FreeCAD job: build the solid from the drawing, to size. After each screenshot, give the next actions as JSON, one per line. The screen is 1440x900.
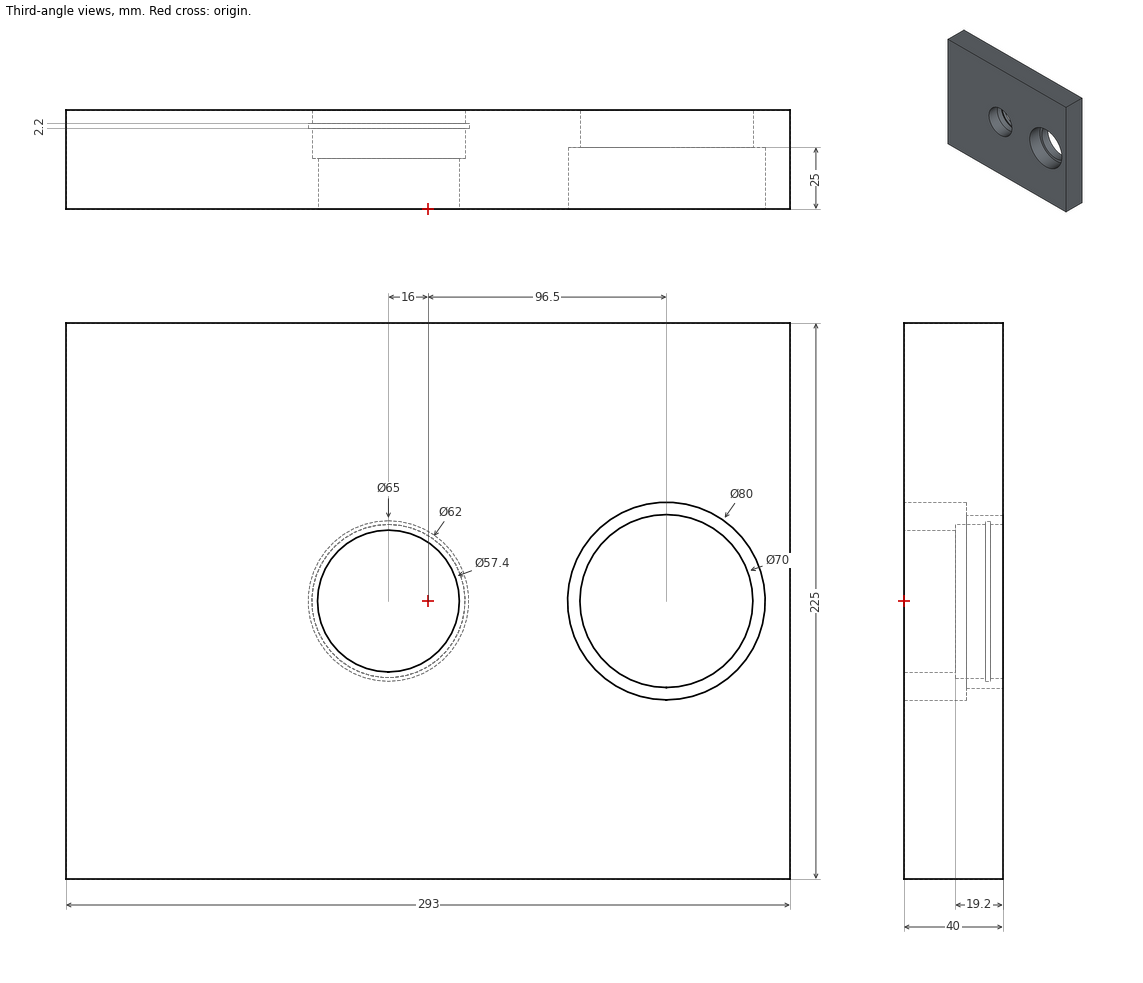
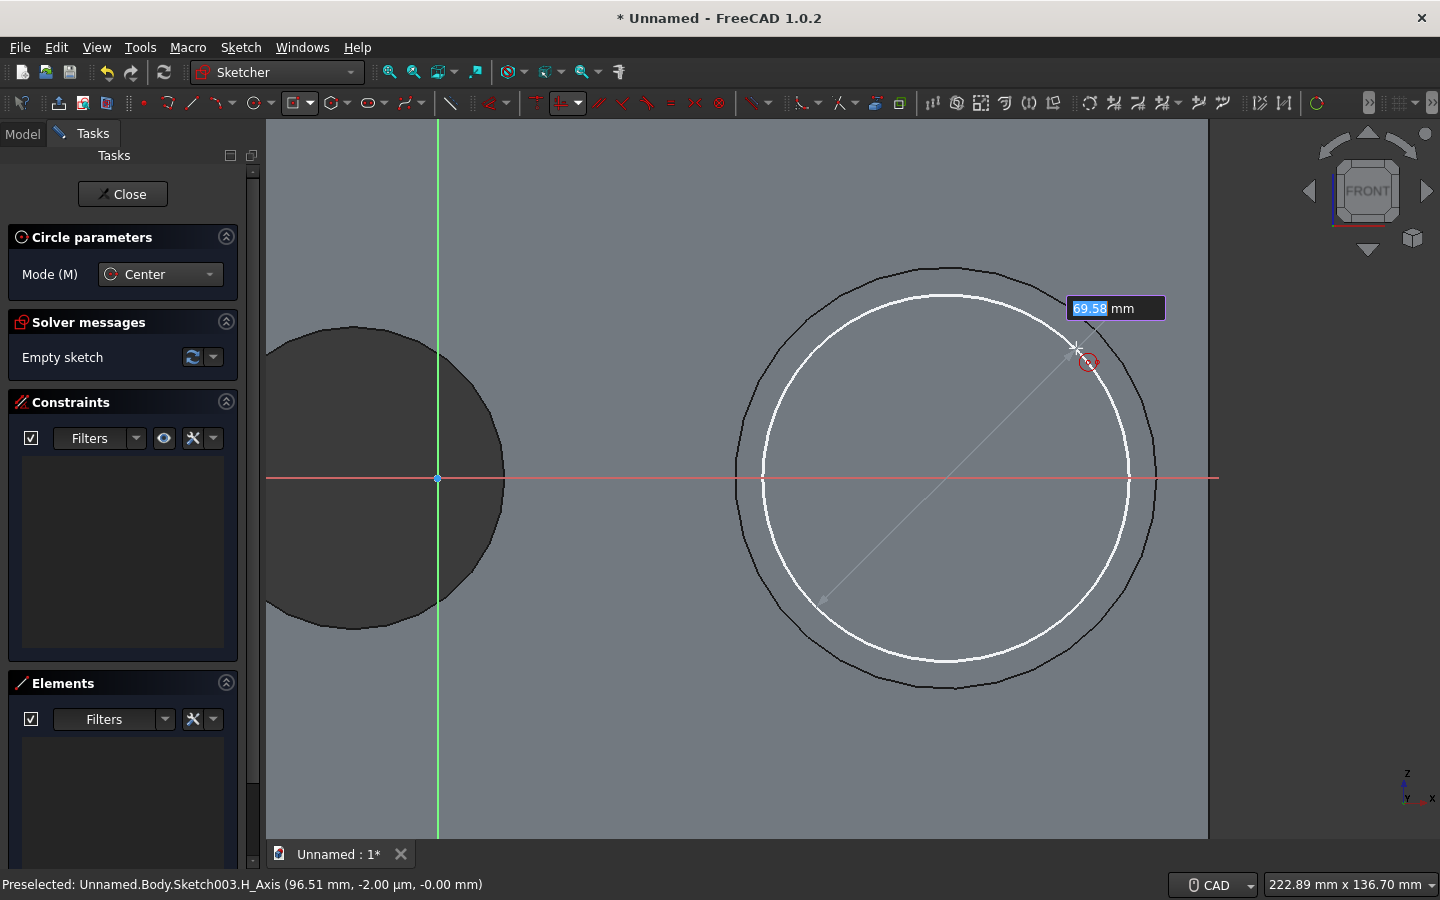
{"action": "type", "text": "70"}
{"action": "key", "text": "Return"}
{"action": "key", "text": "Escape"}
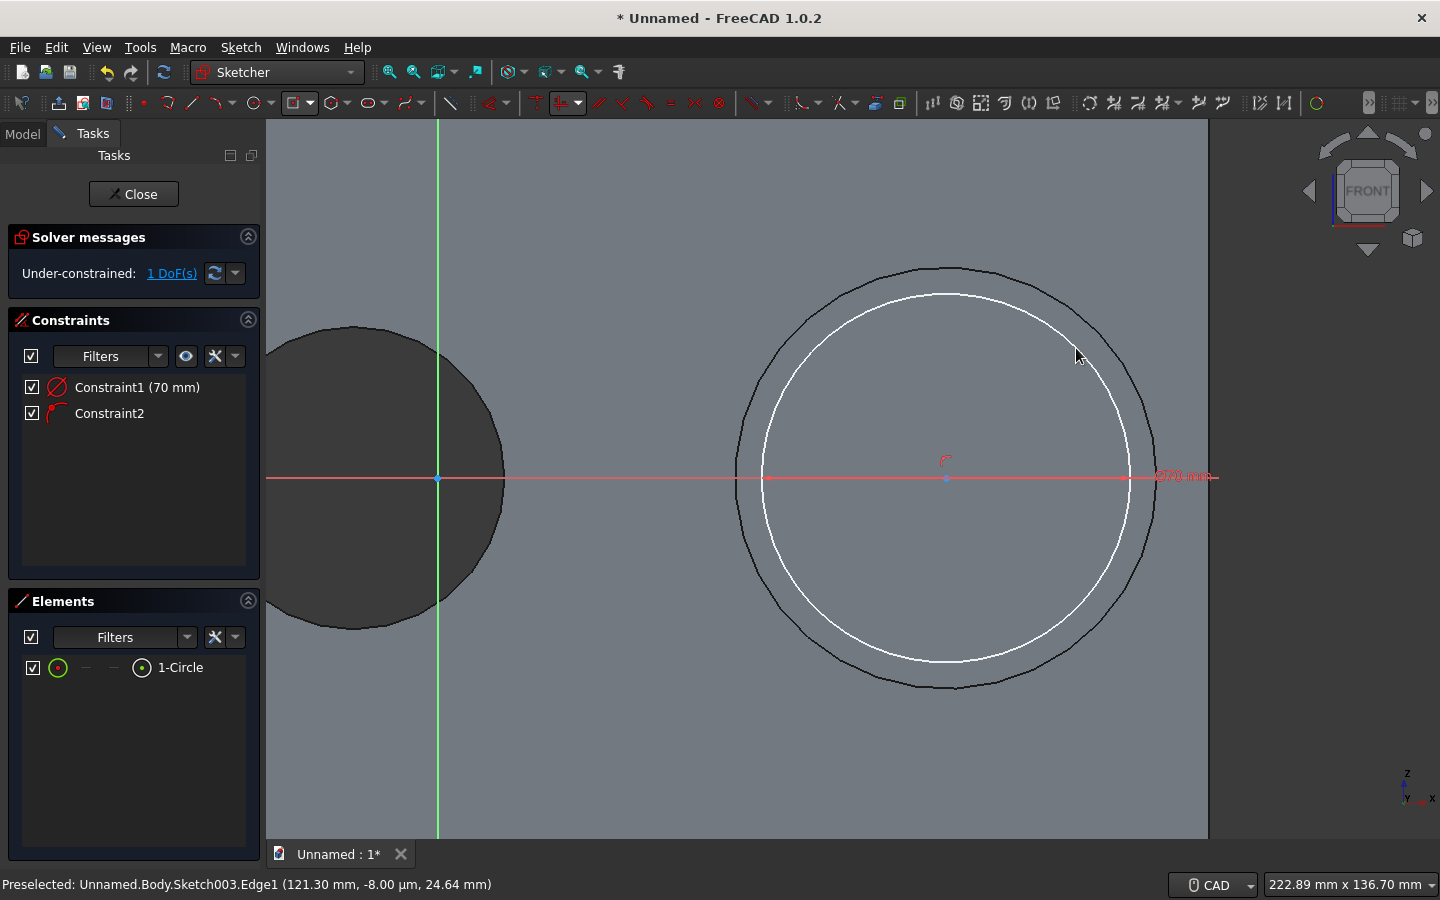
{"action": "left_click", "coordinate": [490, 104]}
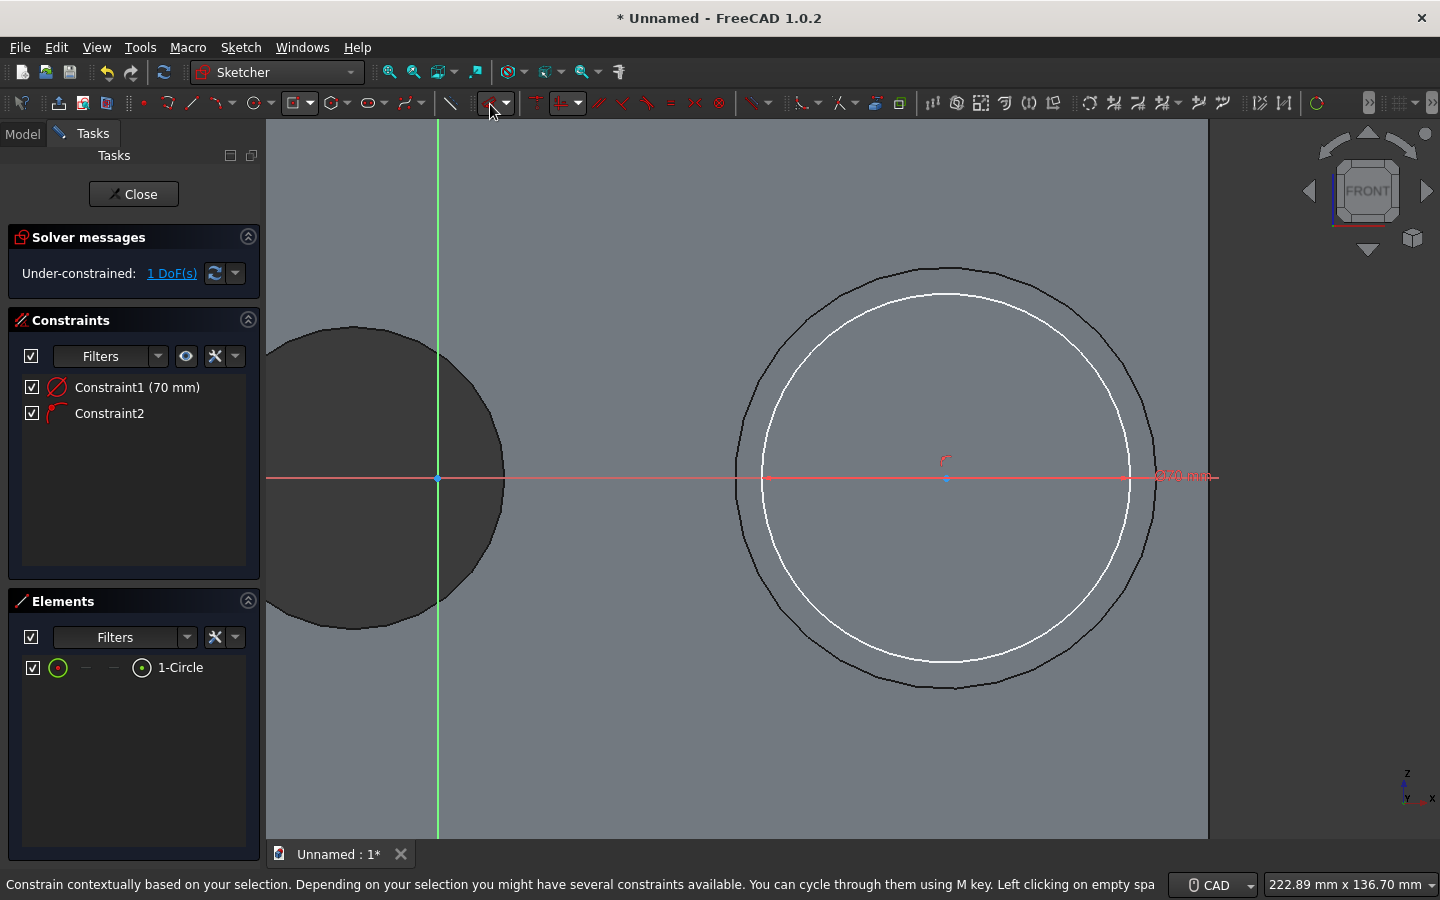
{"action": "left_click", "coordinate": [946, 478]}
{"action": "left_click", "coordinate": [692, 512]}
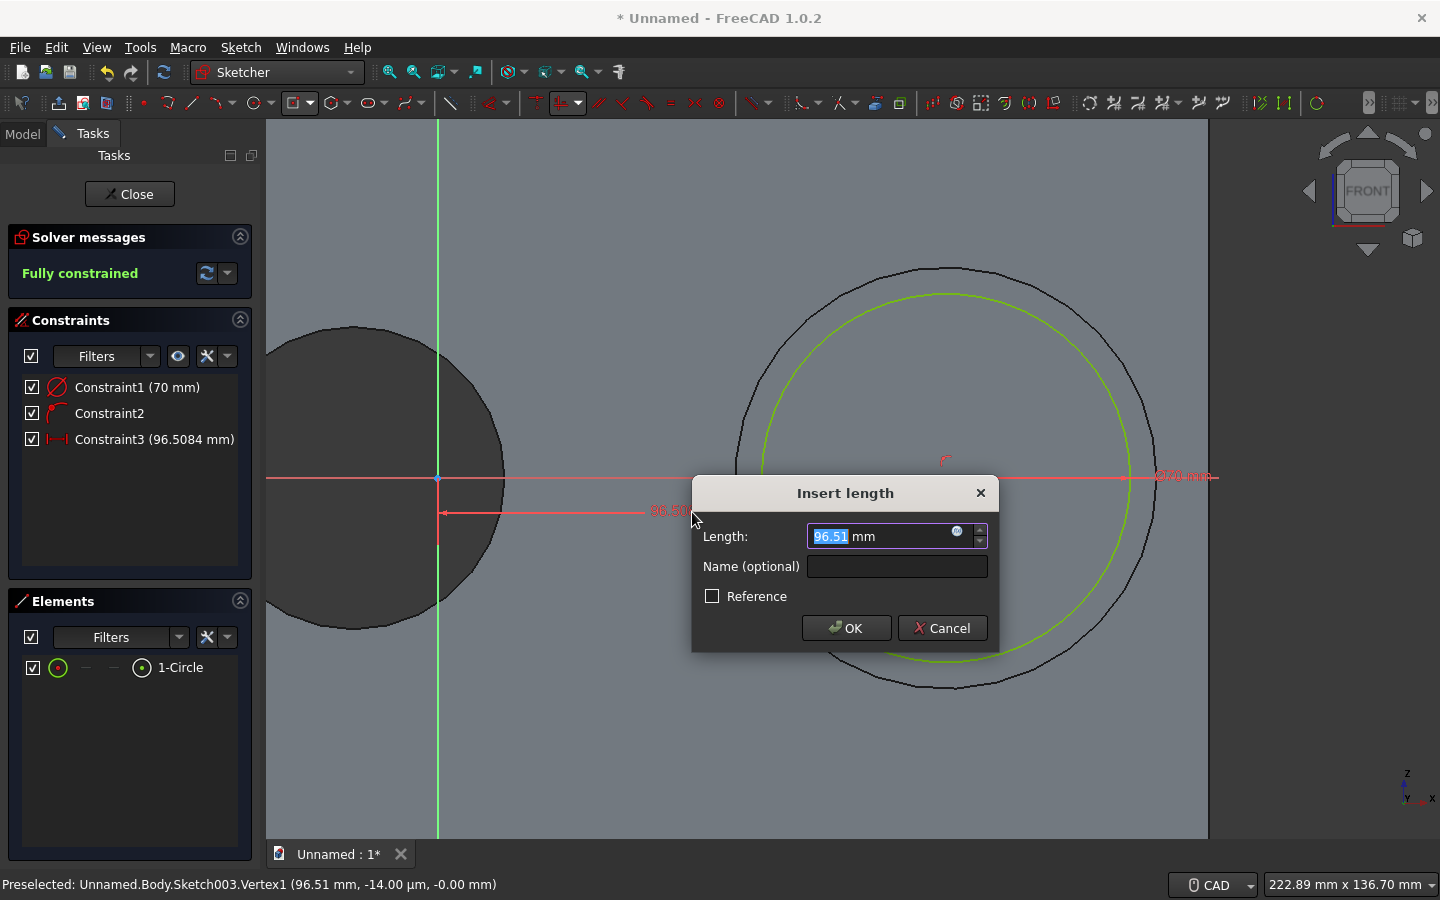
{"action": "type", "text": "96.5"}
{"action": "key", "text": "Return"}
{"action": "key", "text": "Escape"}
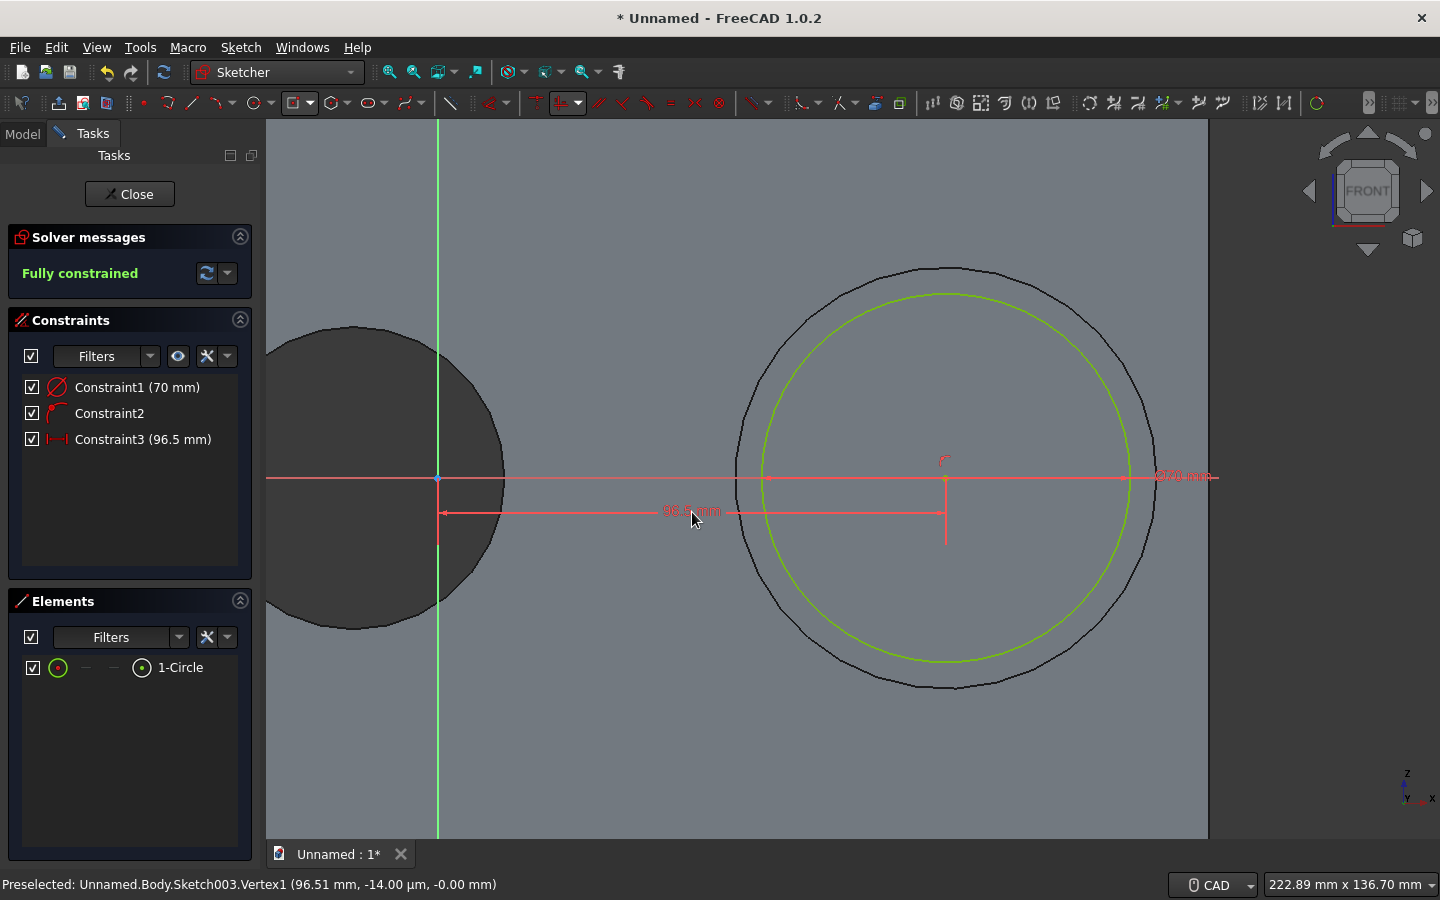
{"action": "left_click", "coordinate": [130, 194]}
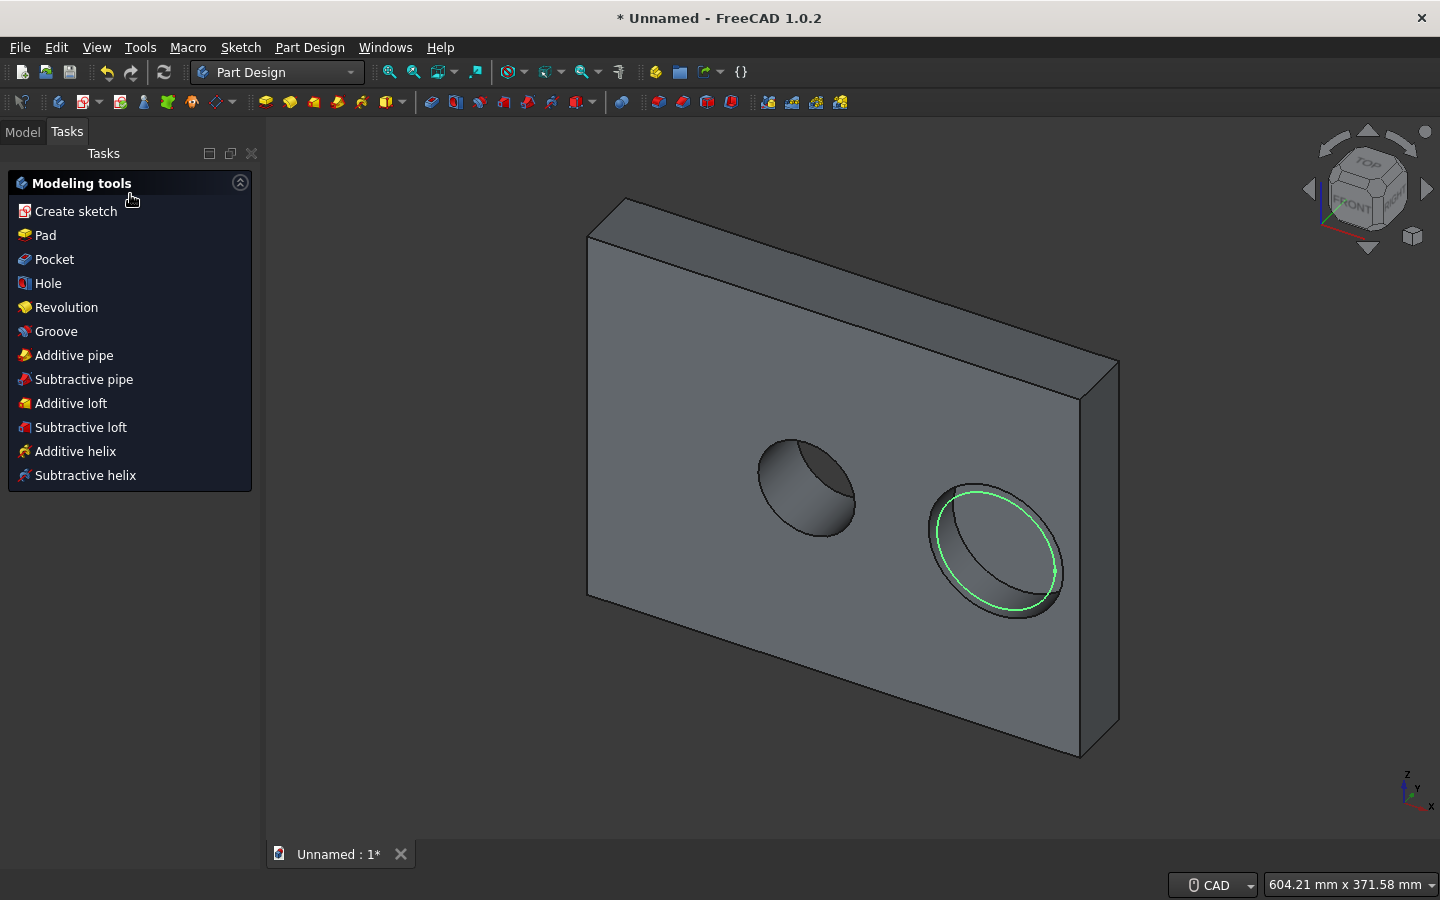
{"action": "left_click", "coordinate": [432, 102]}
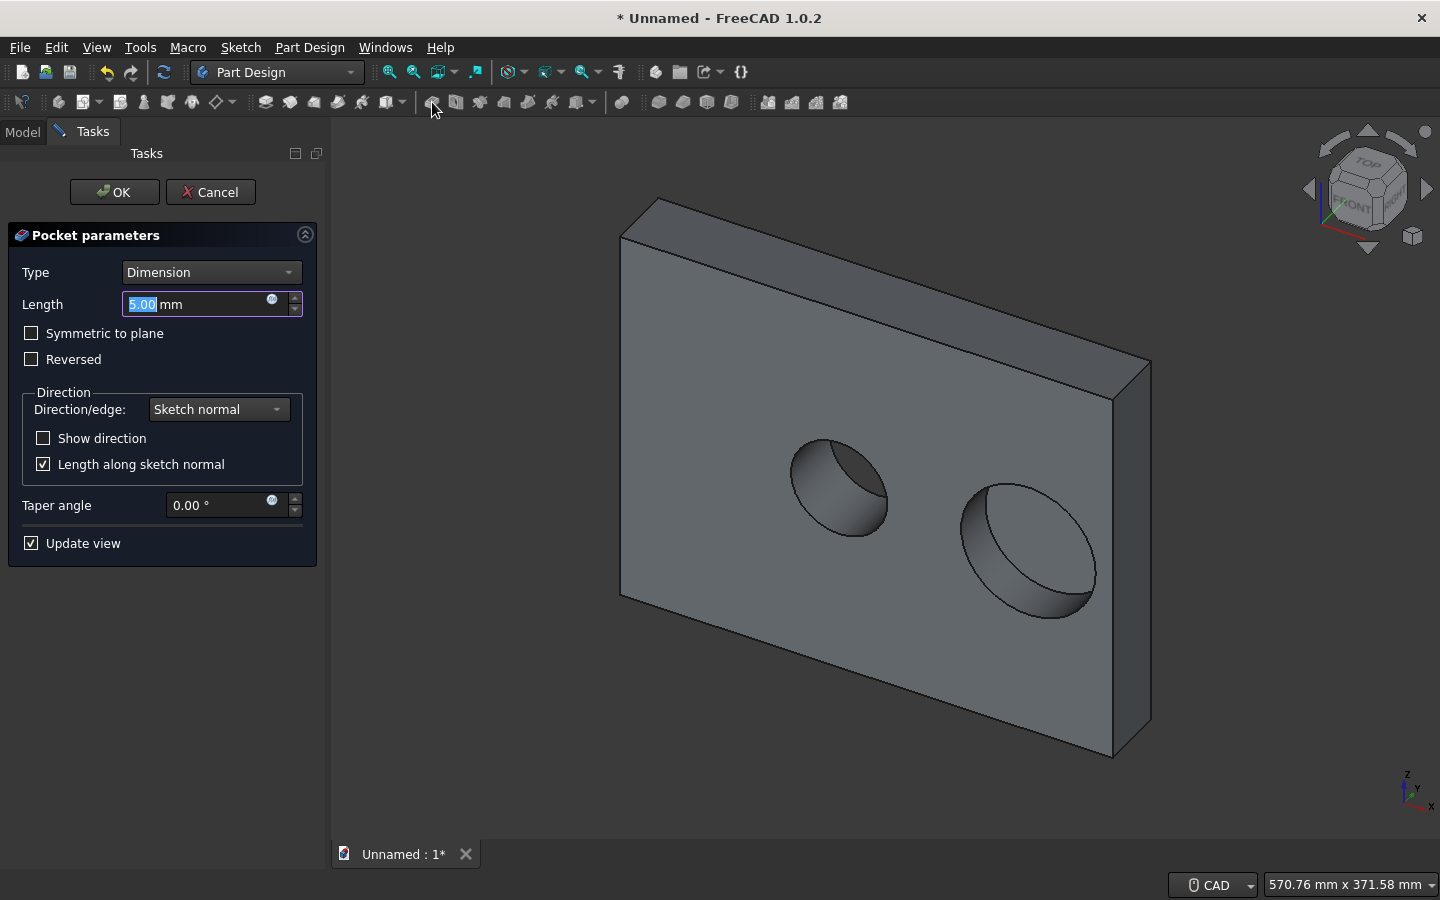
{"action": "left_click", "coordinate": [212, 272]}